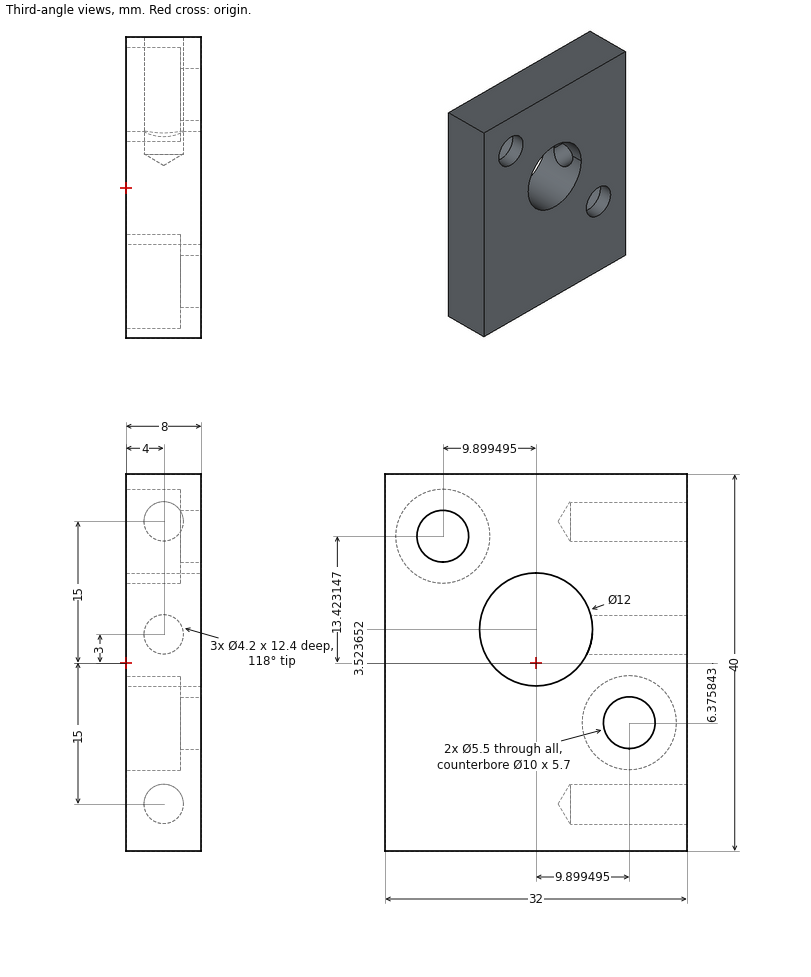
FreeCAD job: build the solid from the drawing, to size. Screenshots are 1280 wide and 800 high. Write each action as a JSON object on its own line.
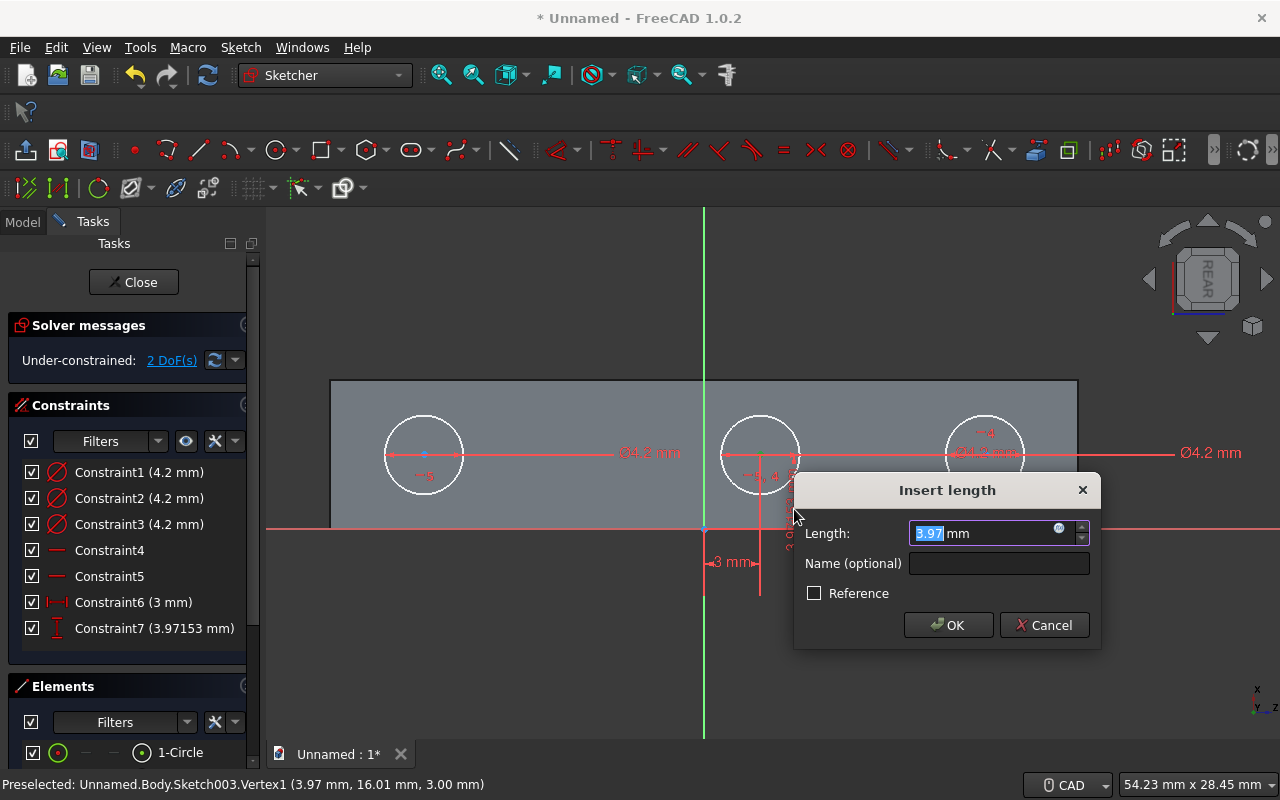
{"action": "type", "text": "4"}
{"action": "key", "text": "Return"}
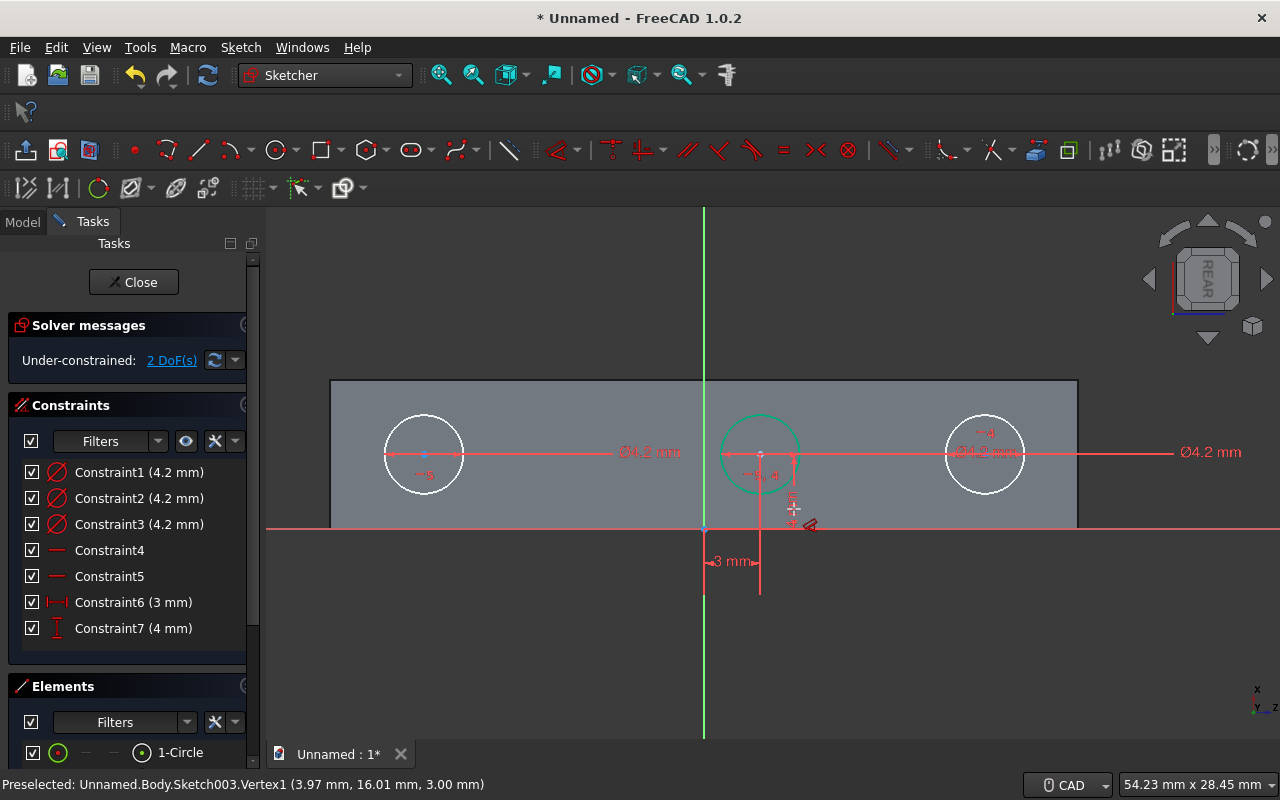
{"action": "left_click", "coordinate": [985, 454]}
{"action": "left_click", "coordinate": [845, 563]}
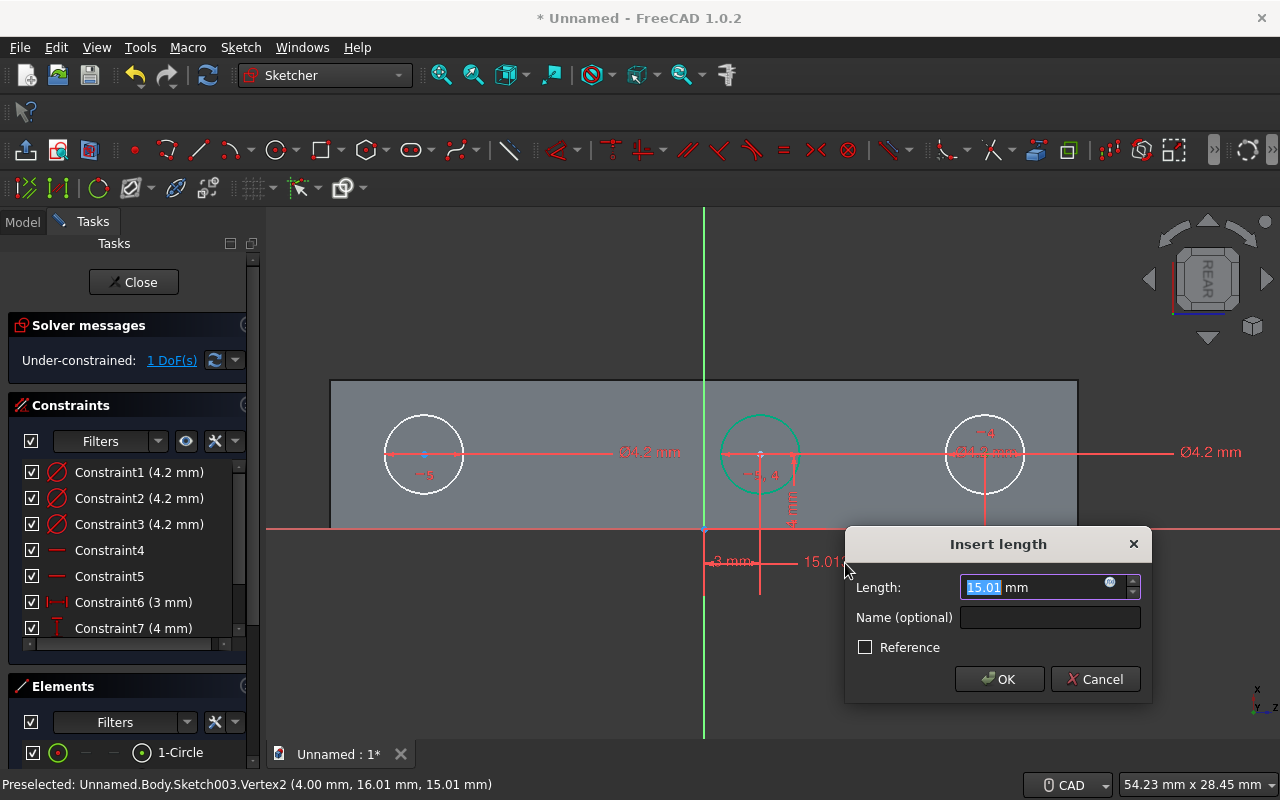
{"action": "type", "text": "15"}
{"action": "key", "text": "Return"}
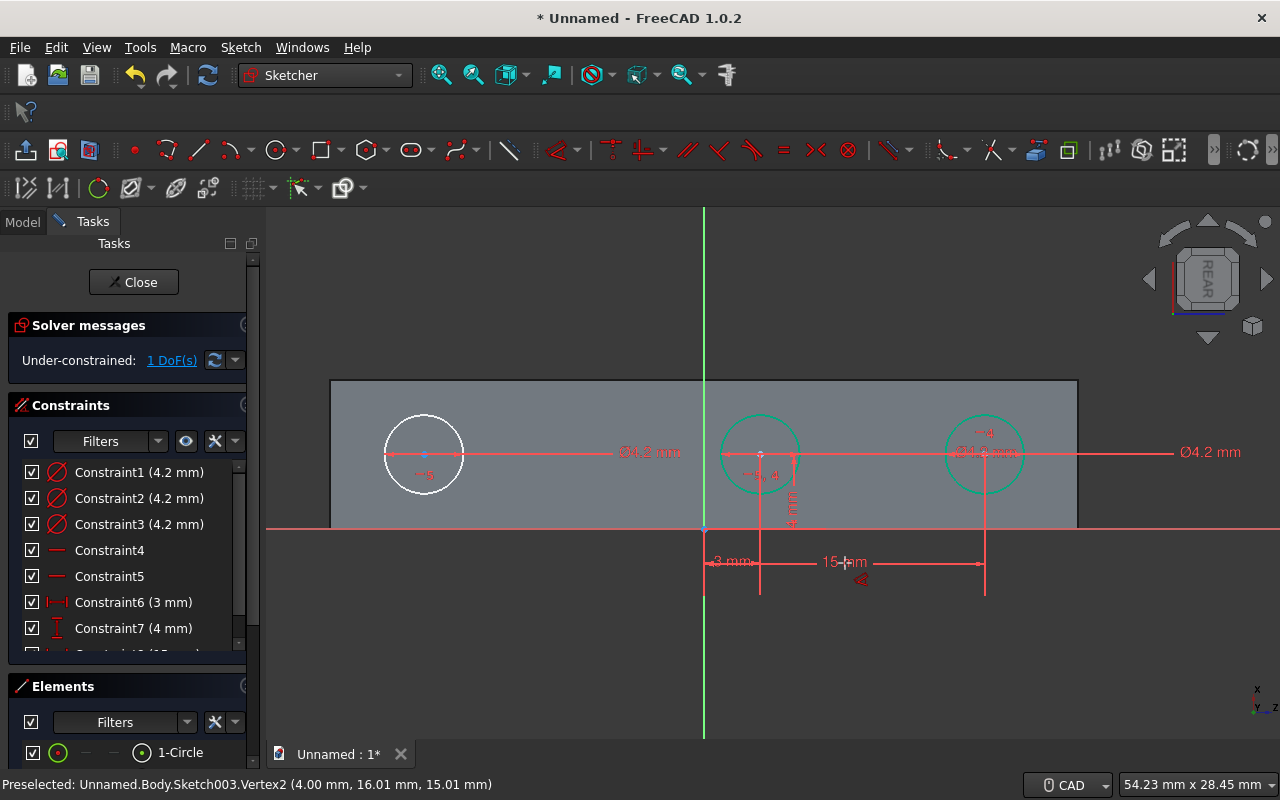
{"action": "left_click", "coordinate": [424, 454]}
{"action": "left_click", "coordinate": [564, 563]}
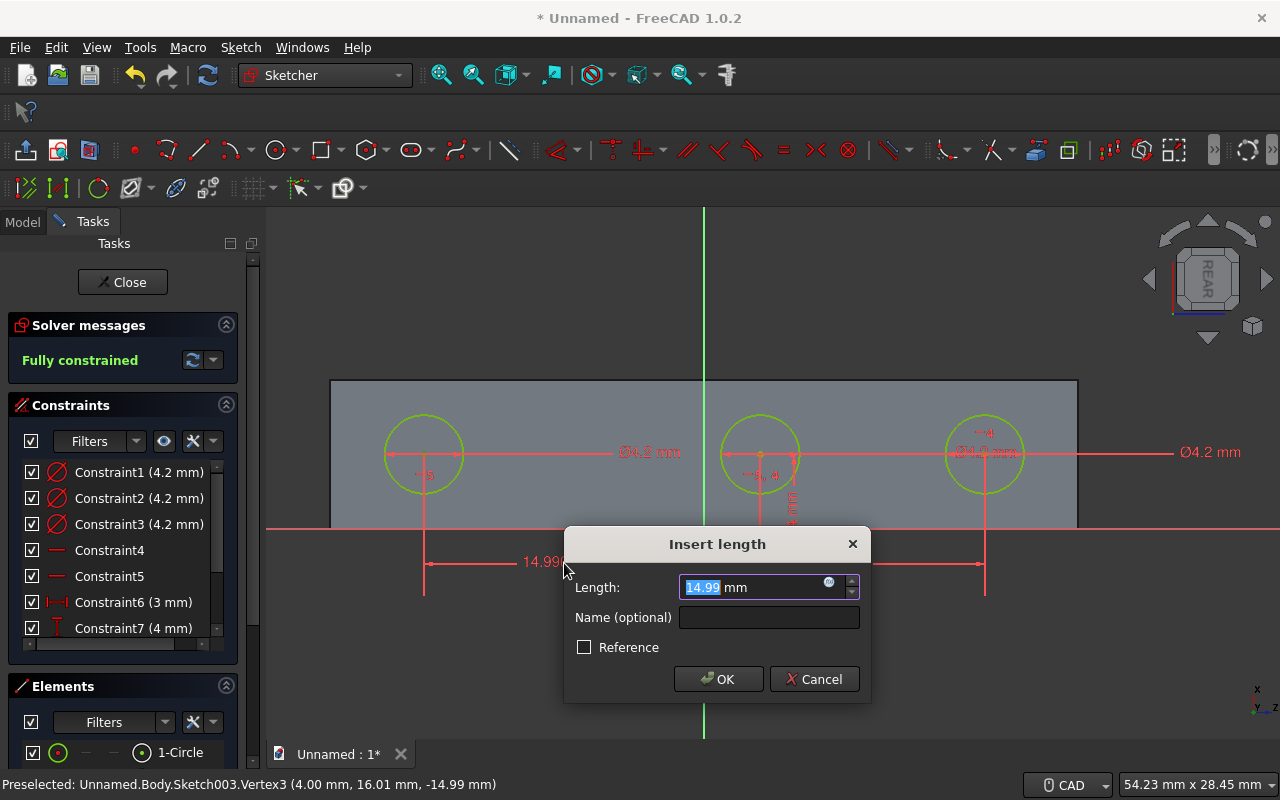
{"action": "type", "text": "15"}
{"action": "key", "text": "Return"}
{"action": "key", "text": "Escape"}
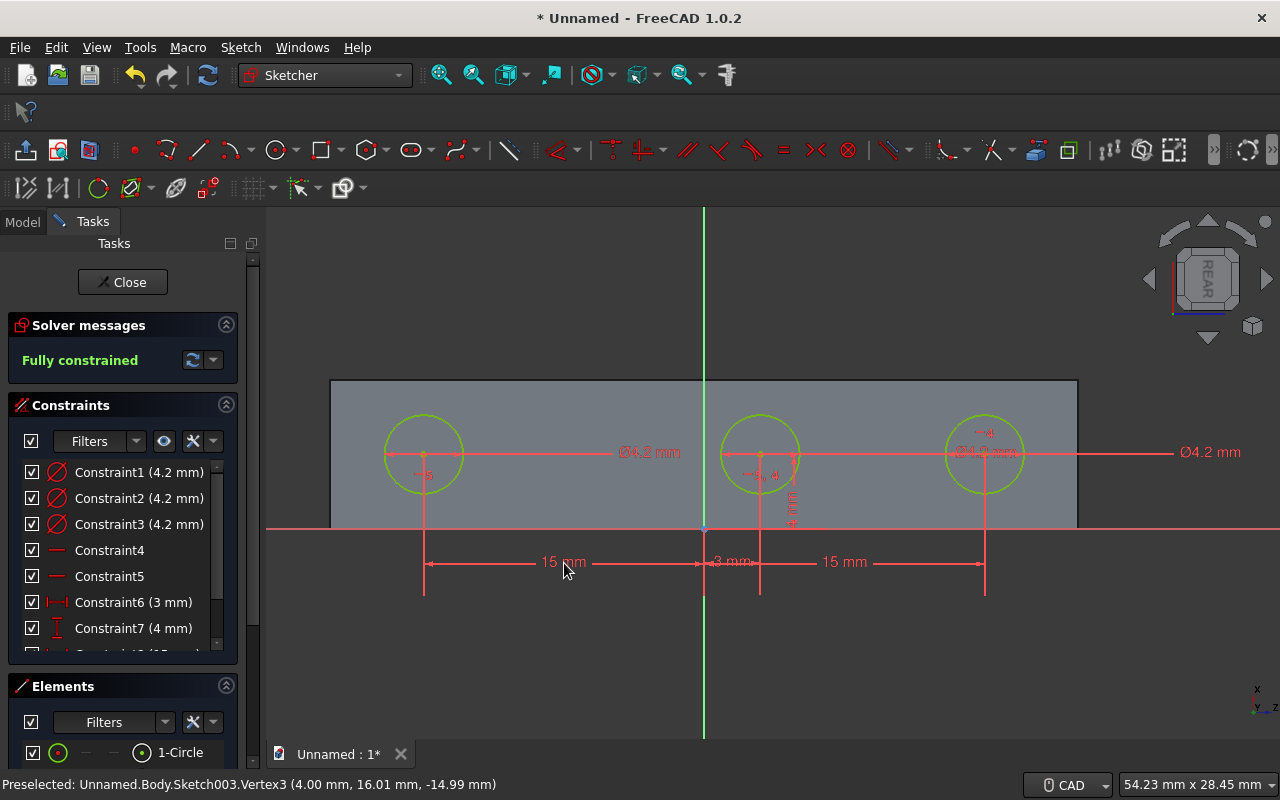
{"action": "left_click", "coordinate": [123, 282]}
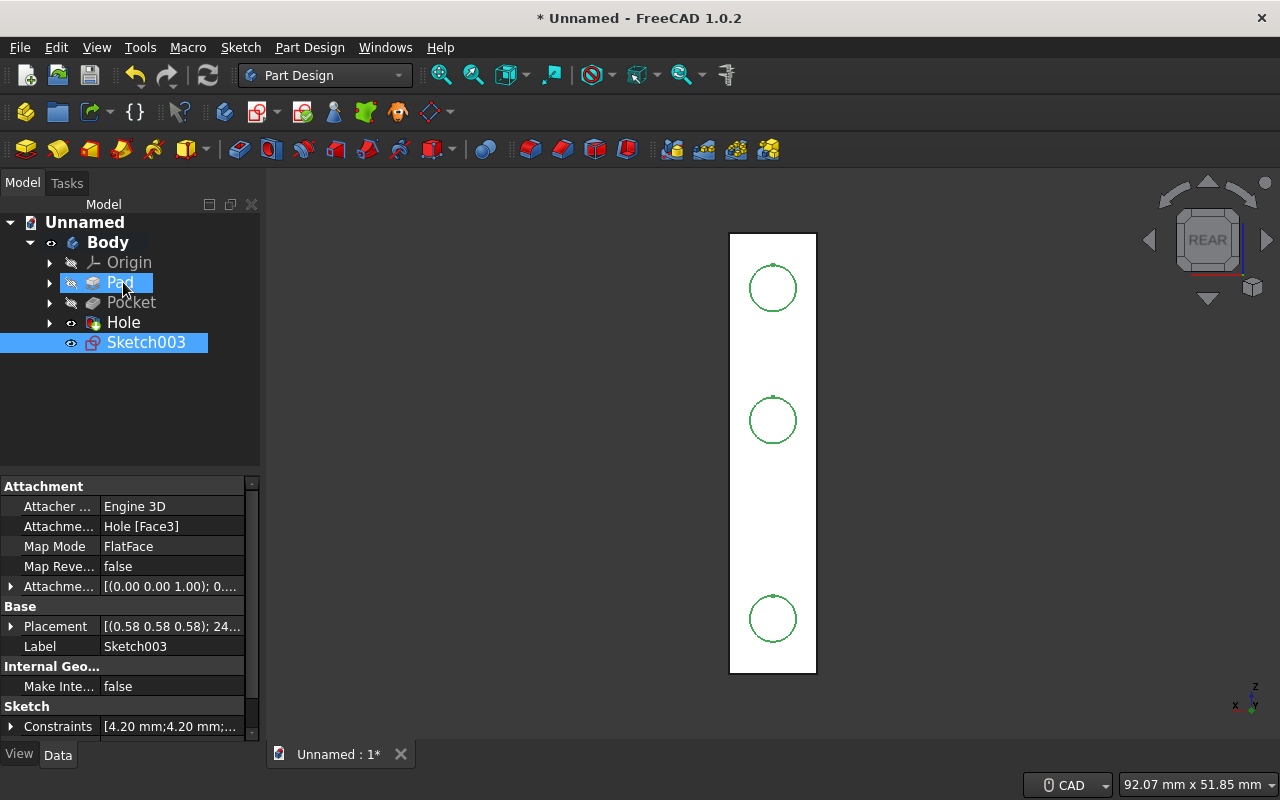
{"action": "left_click", "coordinate": [272, 150]}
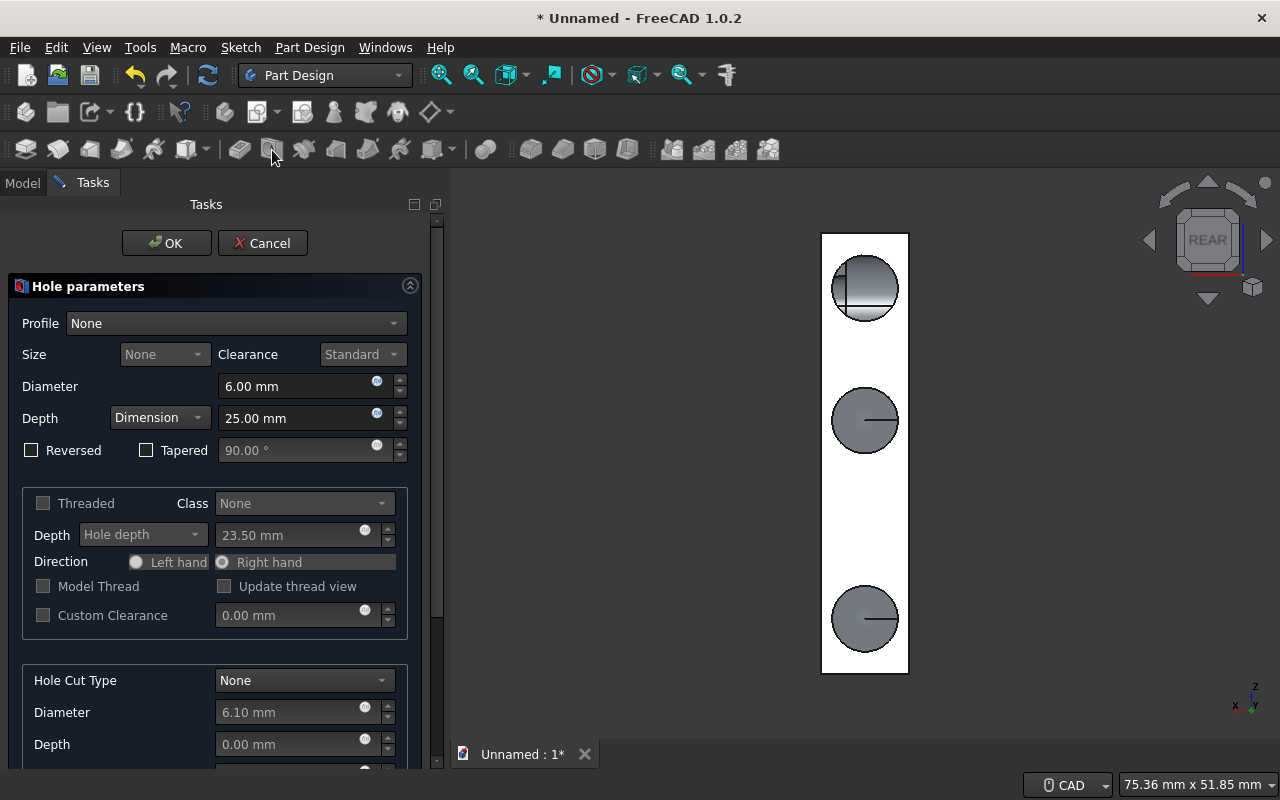
{"action": "triple_click", "coordinate": [305, 386]}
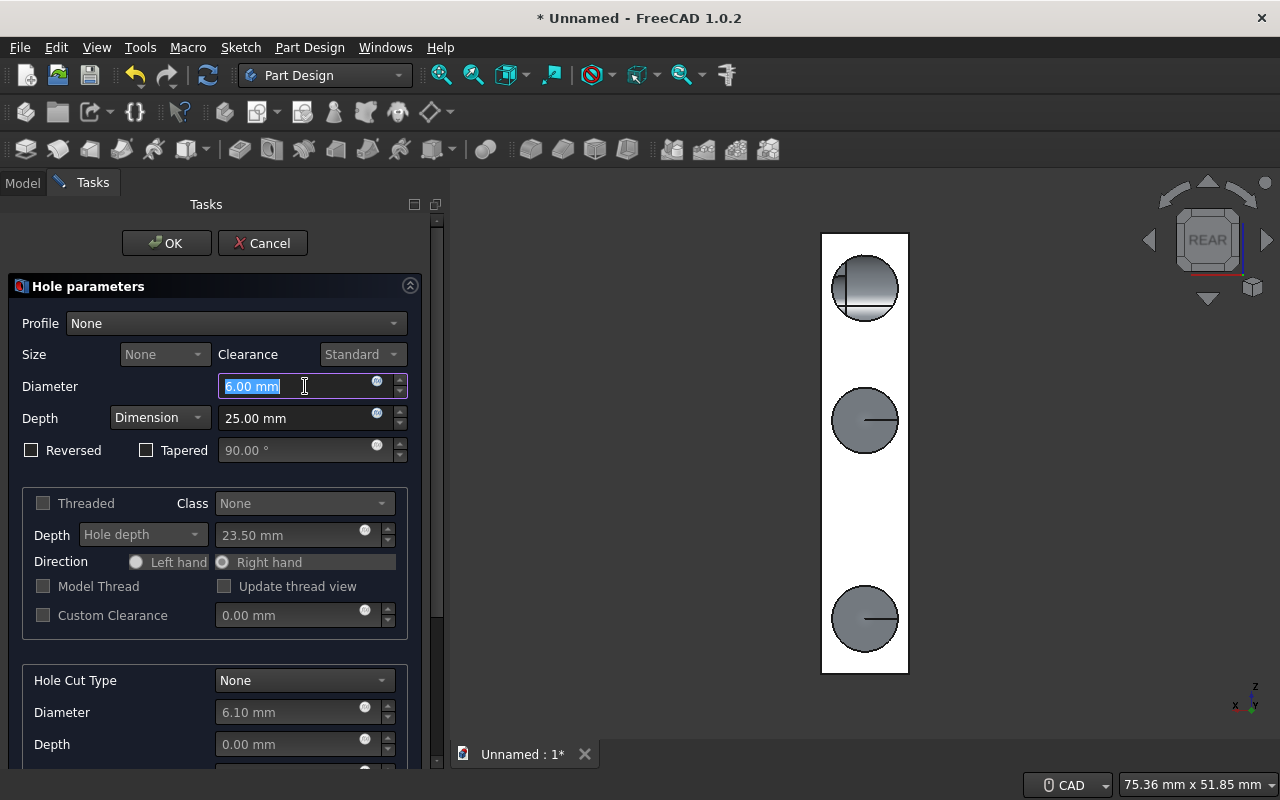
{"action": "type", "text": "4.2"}
{"action": "key", "text": "Tab"}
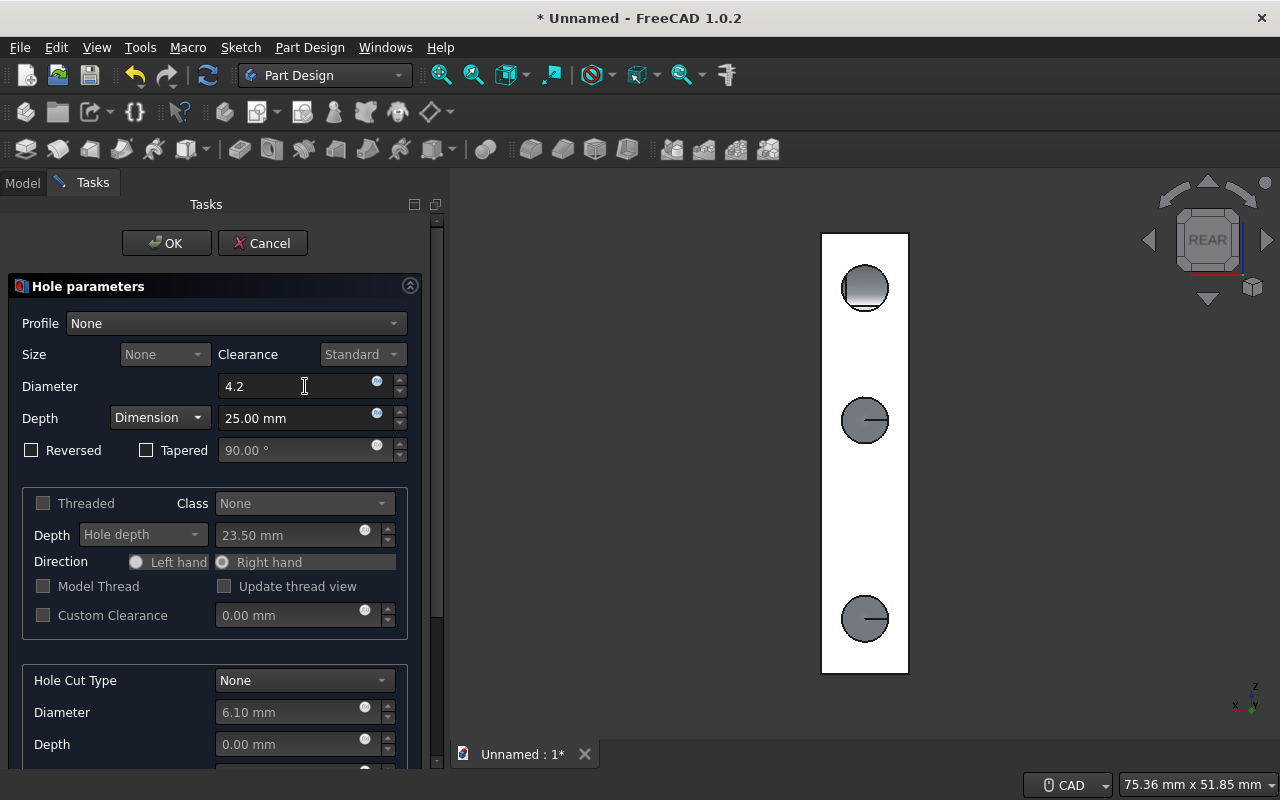
{"action": "triple_click", "coordinate": [305, 418]}